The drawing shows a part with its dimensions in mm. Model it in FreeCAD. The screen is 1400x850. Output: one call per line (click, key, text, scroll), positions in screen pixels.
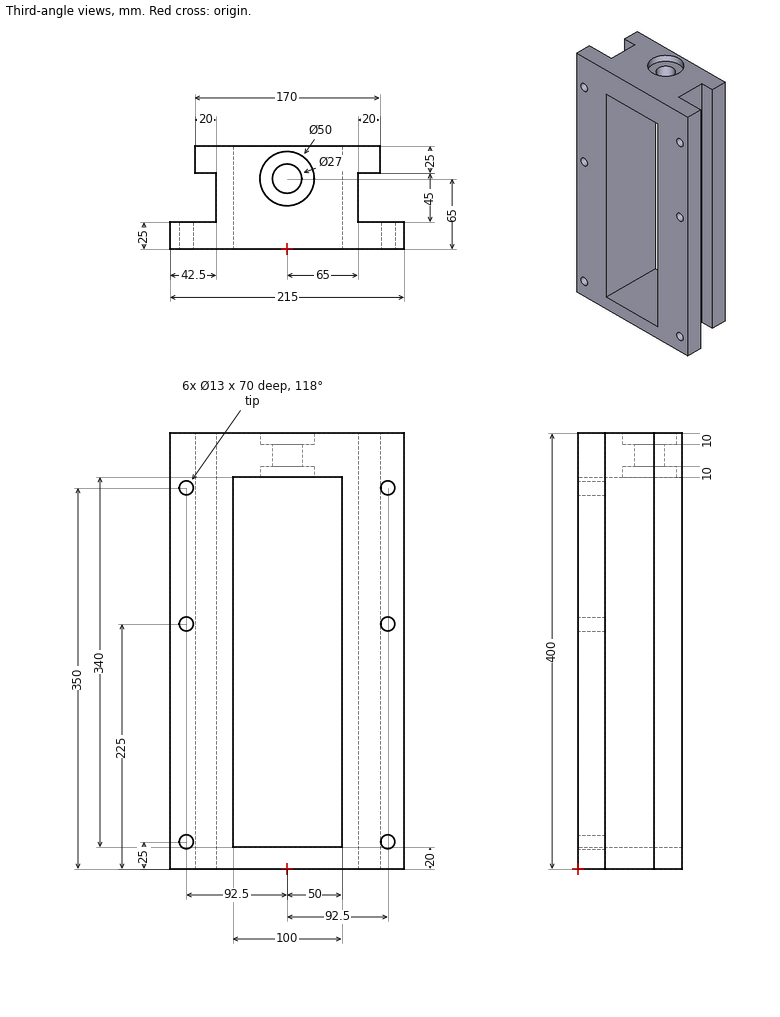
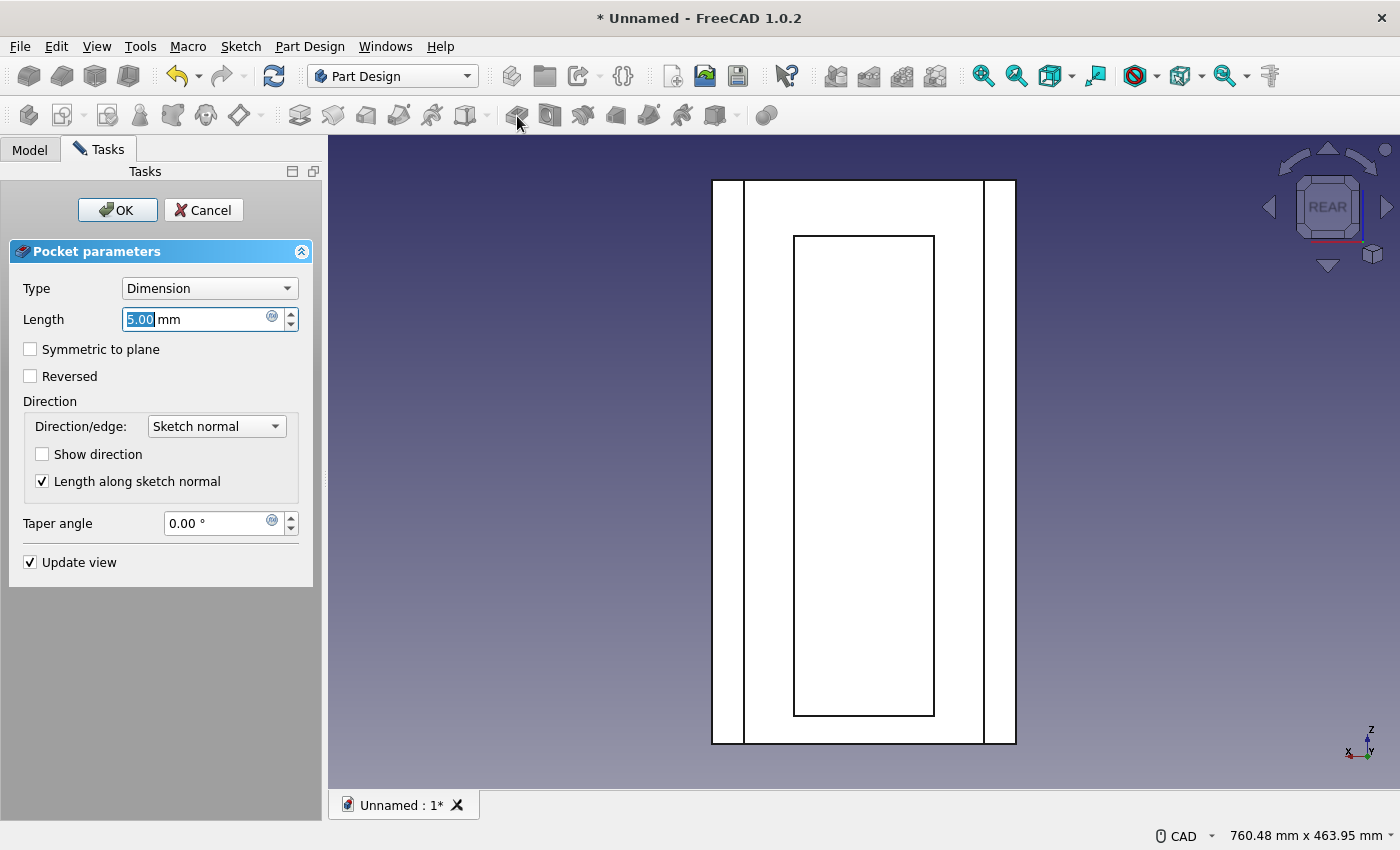
click(210, 288)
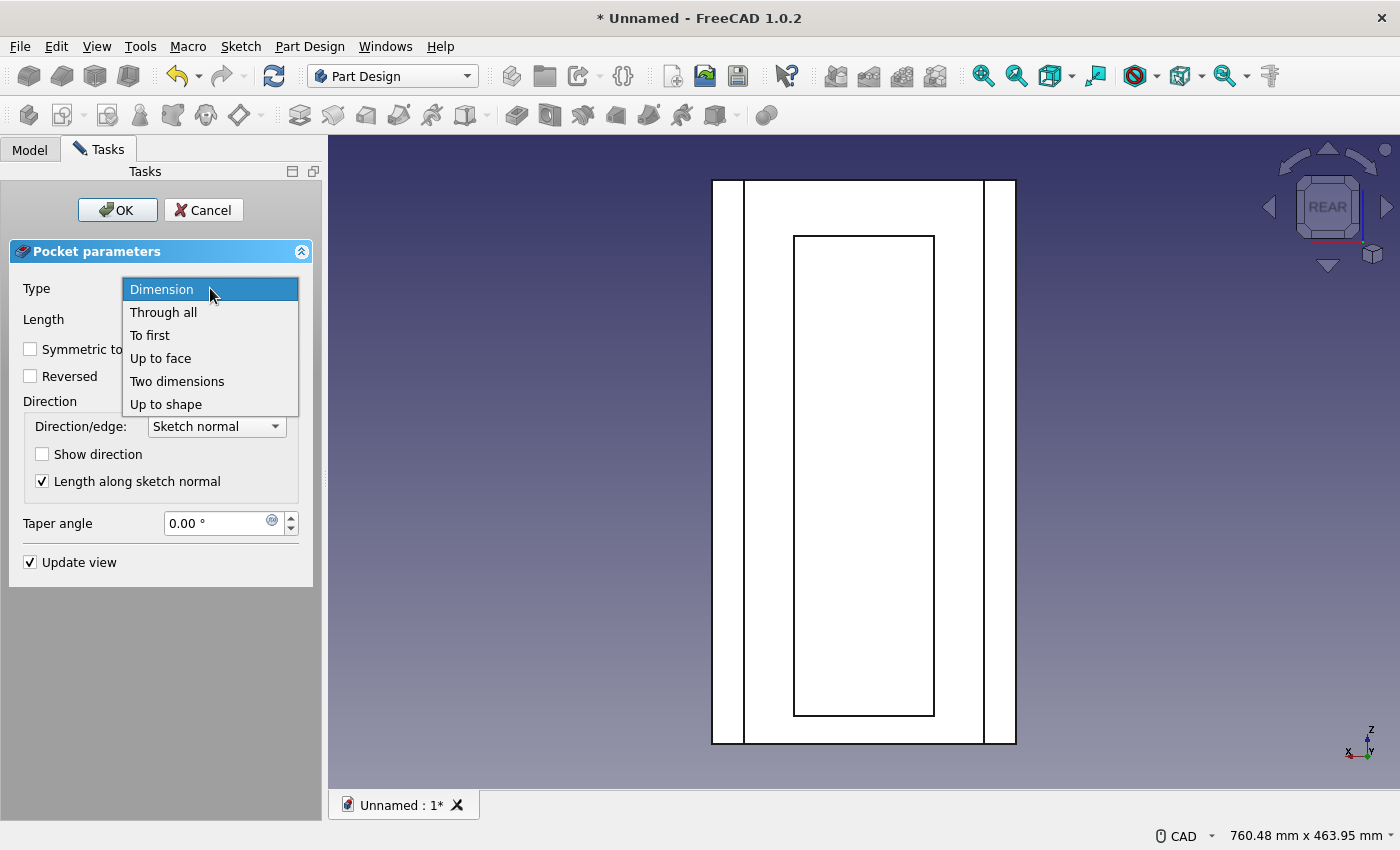
click(208, 336)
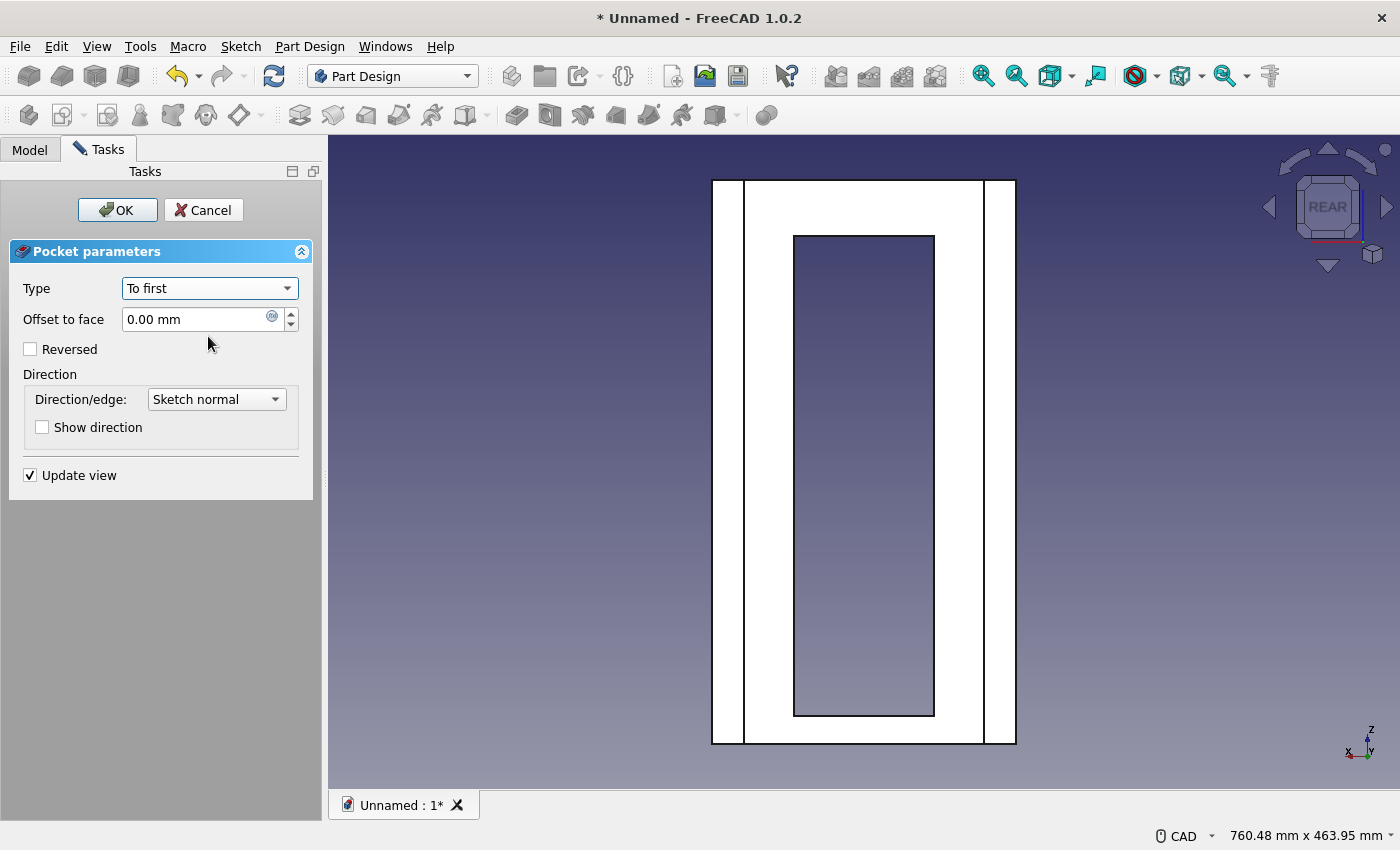
click(118, 210)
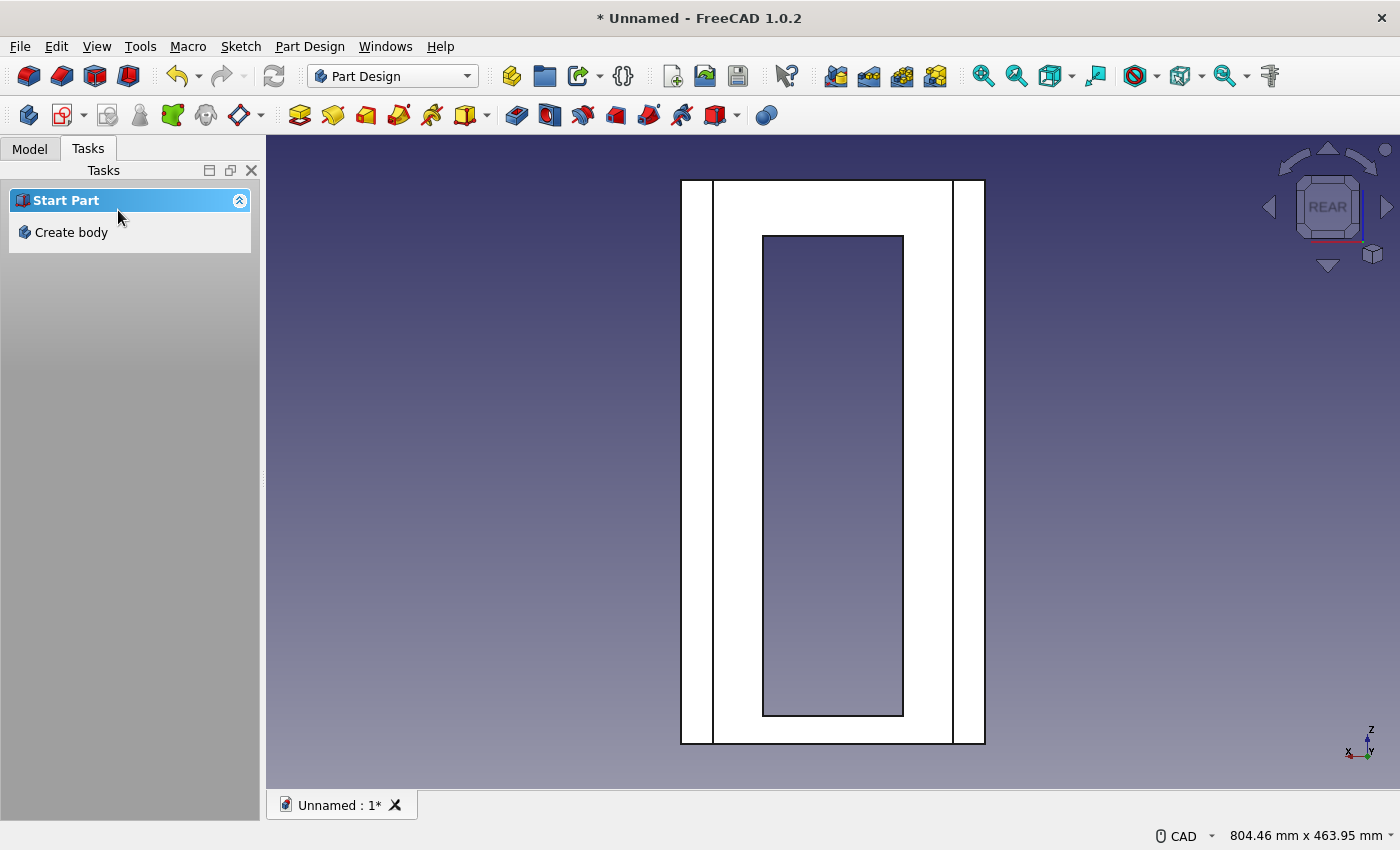
key(0)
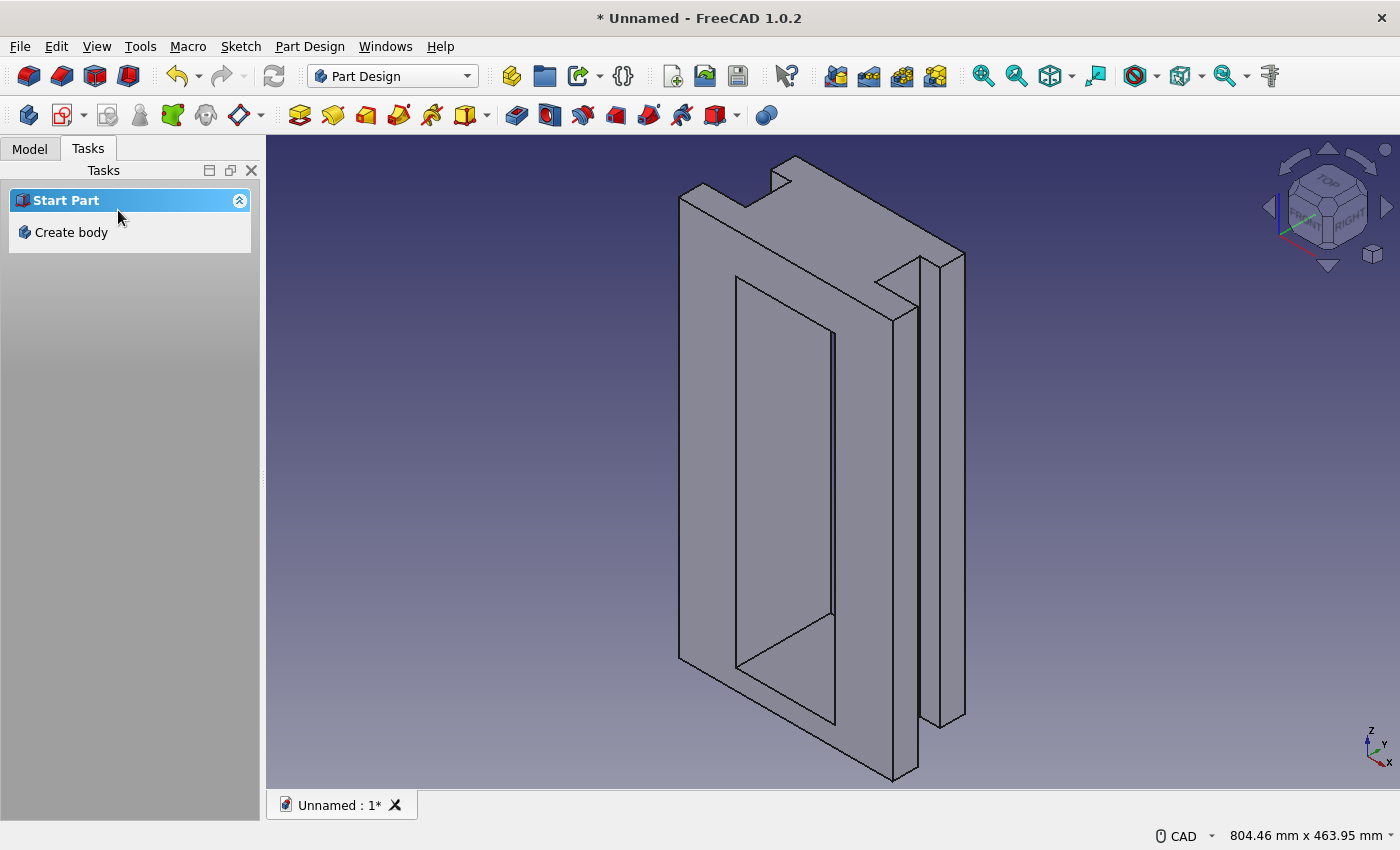
click(833, 231)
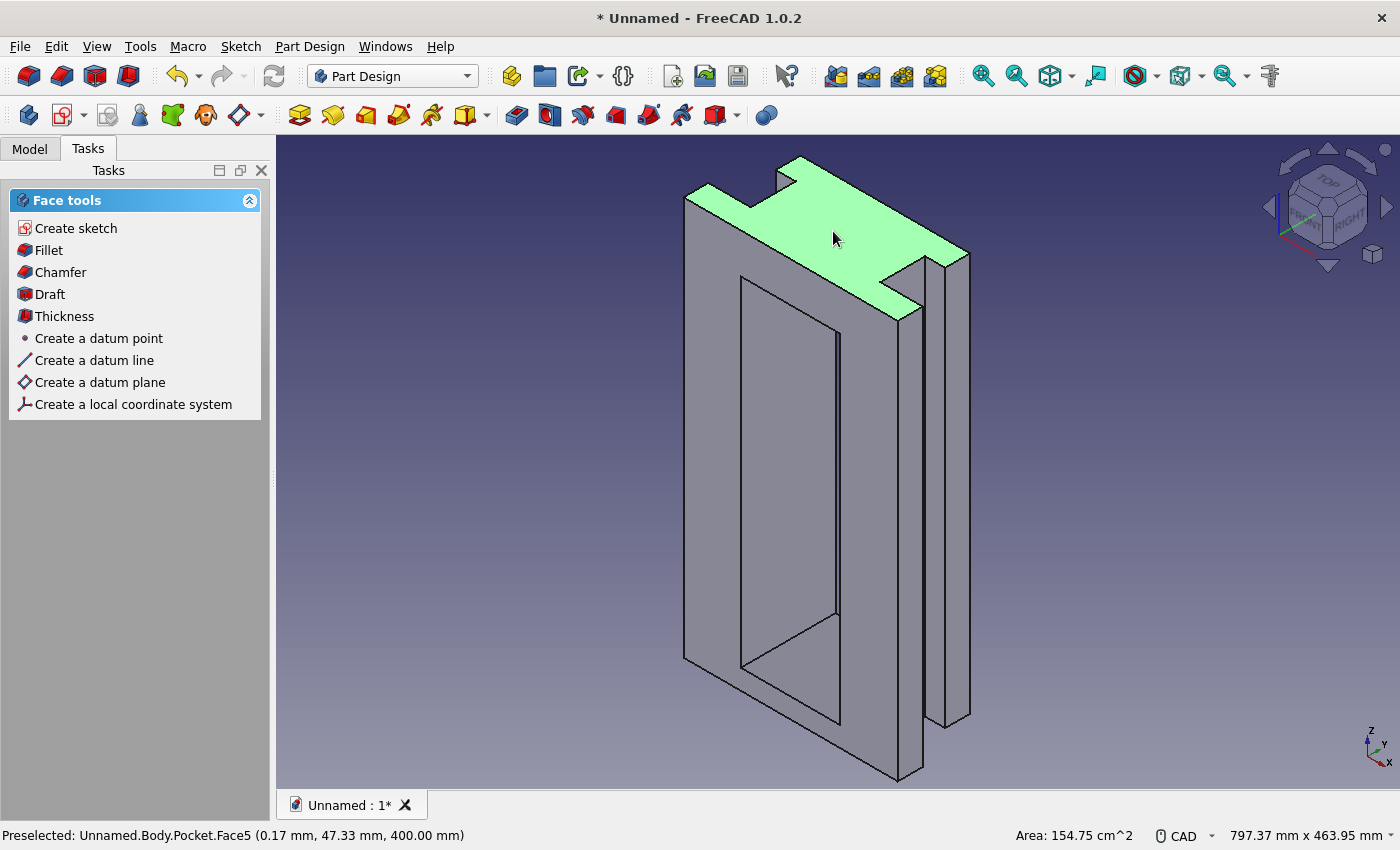
click(62, 116)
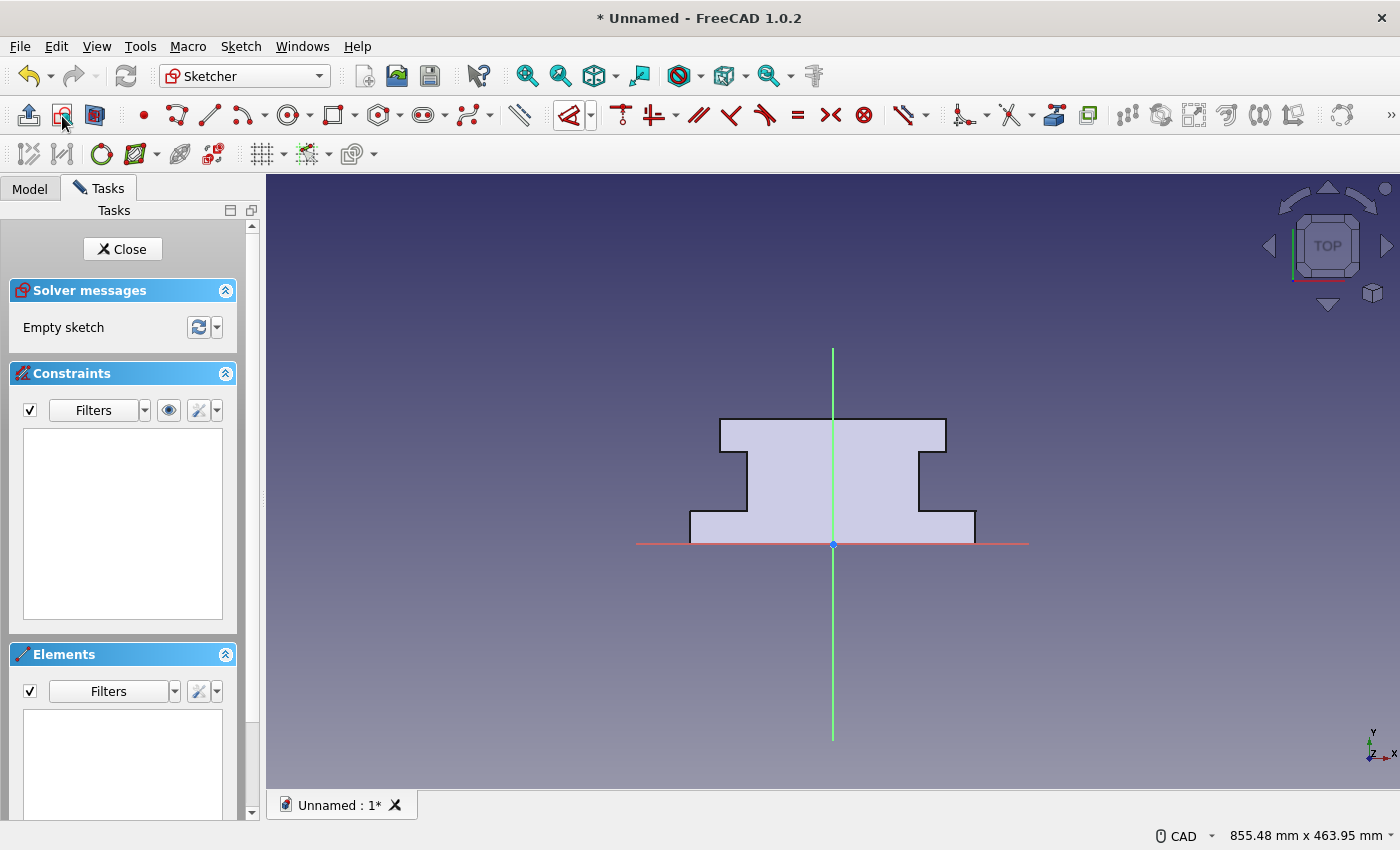
scroll(840, 456, up, 12)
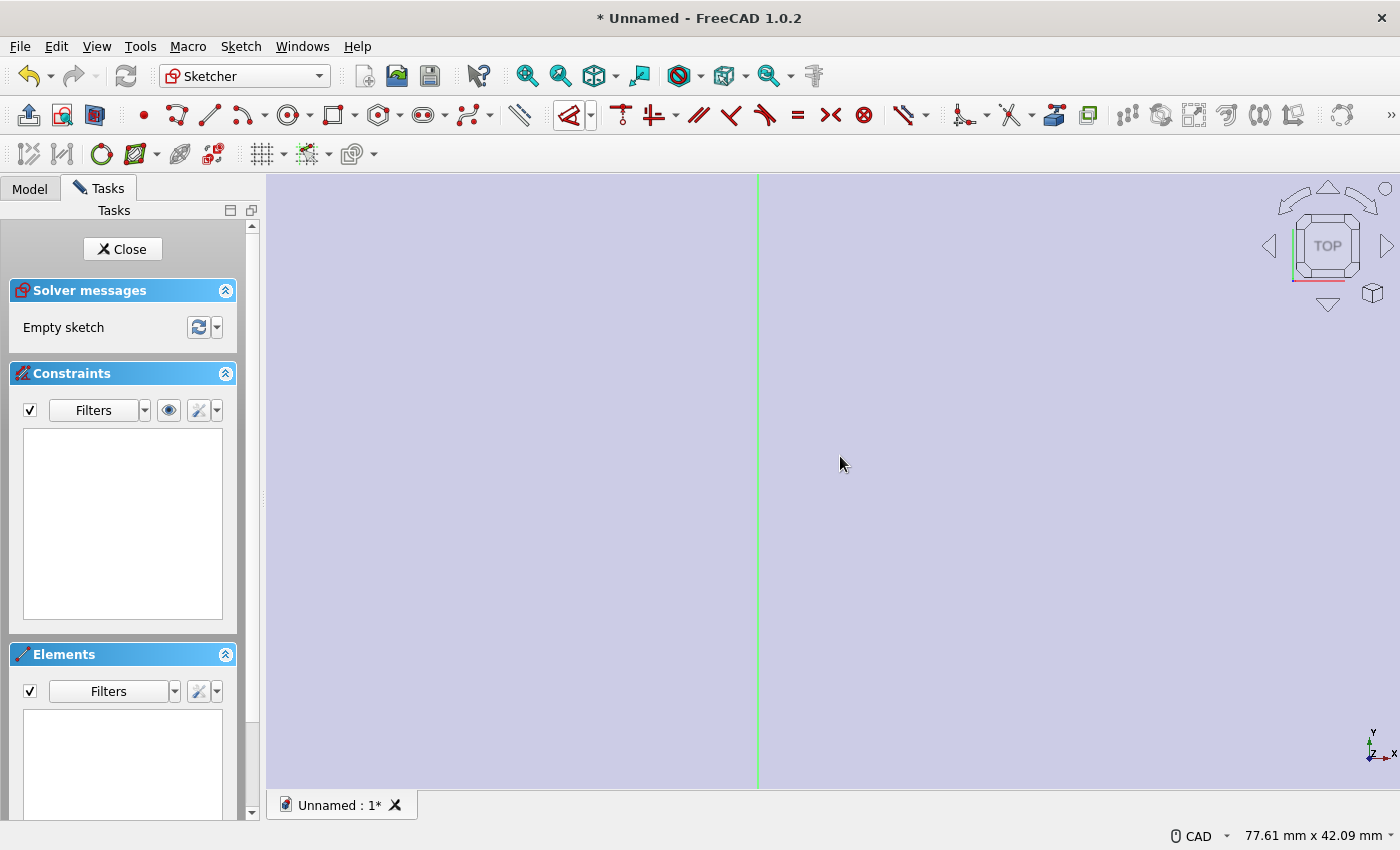
key(g)
key(c)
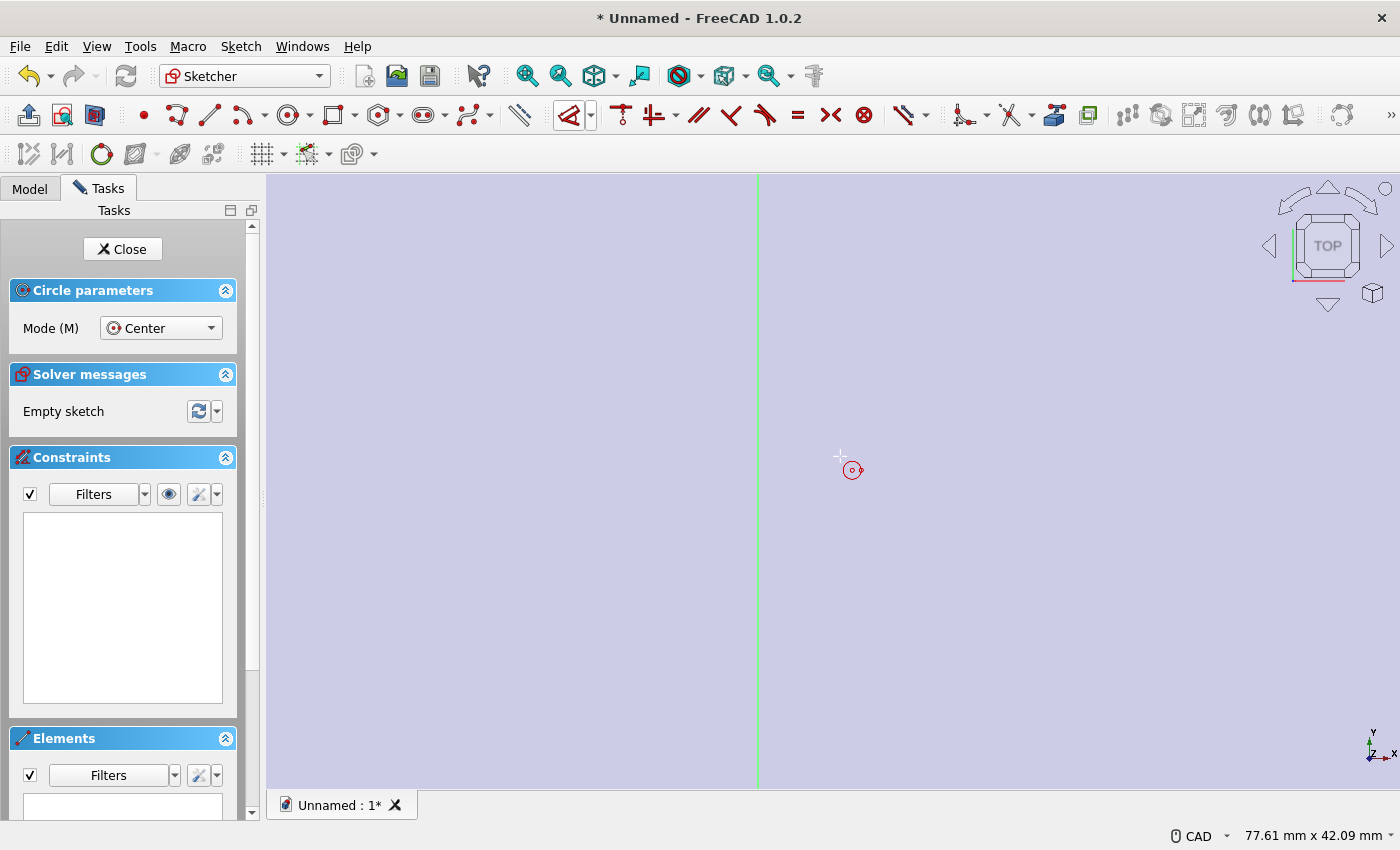
click(758, 477)
move(897, 337)